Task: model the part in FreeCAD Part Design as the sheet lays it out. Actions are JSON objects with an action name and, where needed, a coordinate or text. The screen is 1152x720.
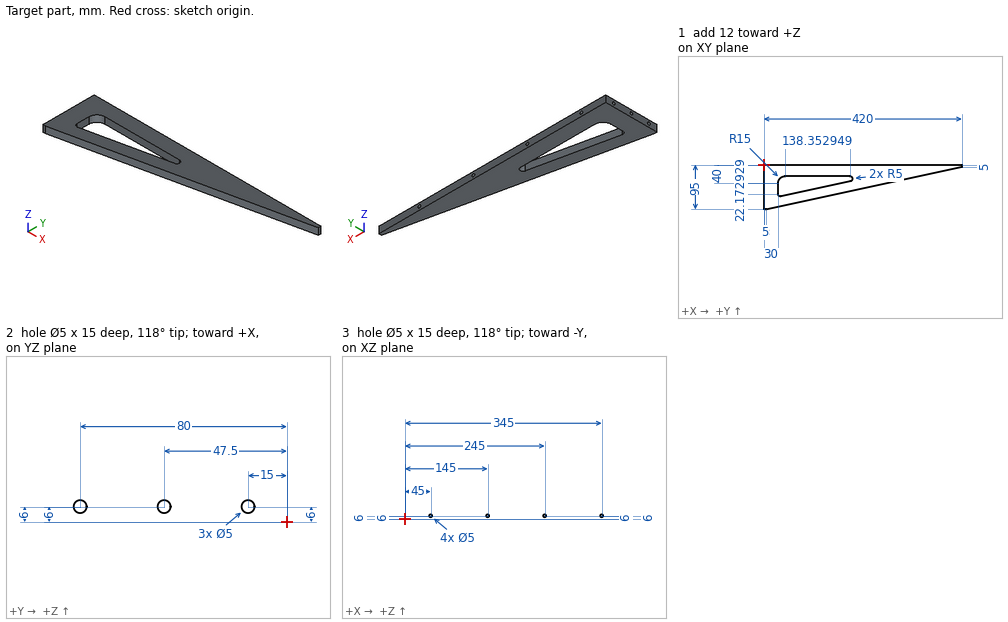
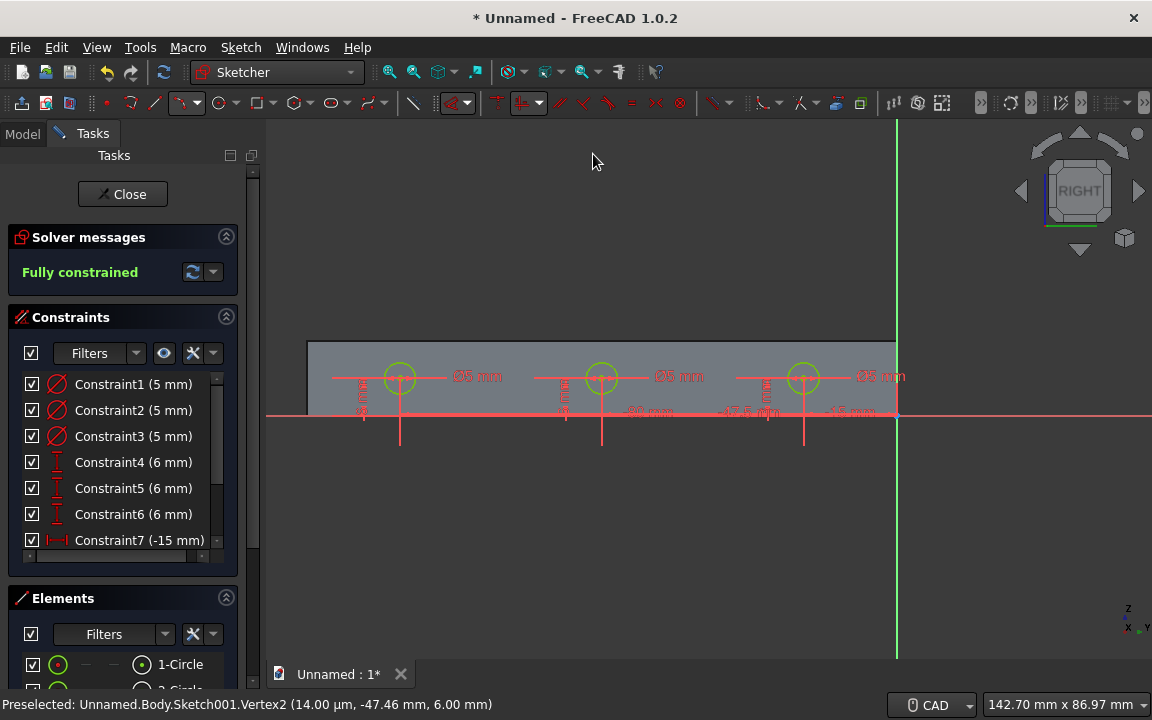
{"action": "left_click", "coordinate": [123, 194]}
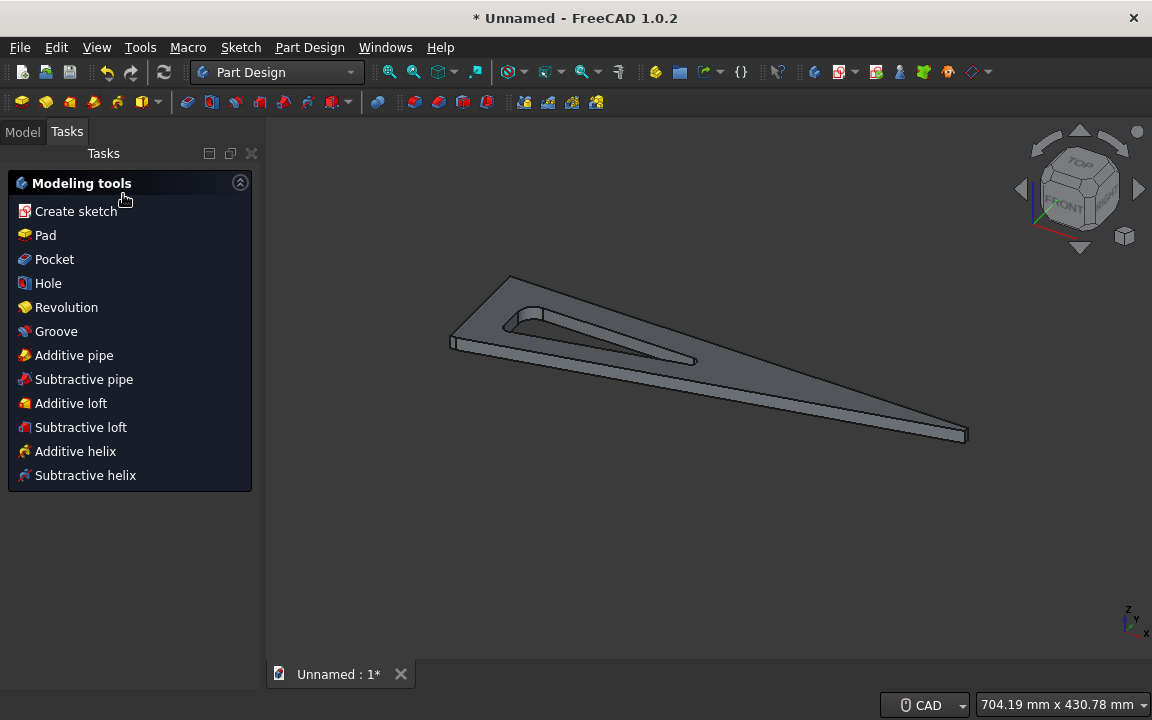
{"action": "left_click", "coordinate": [212, 102]}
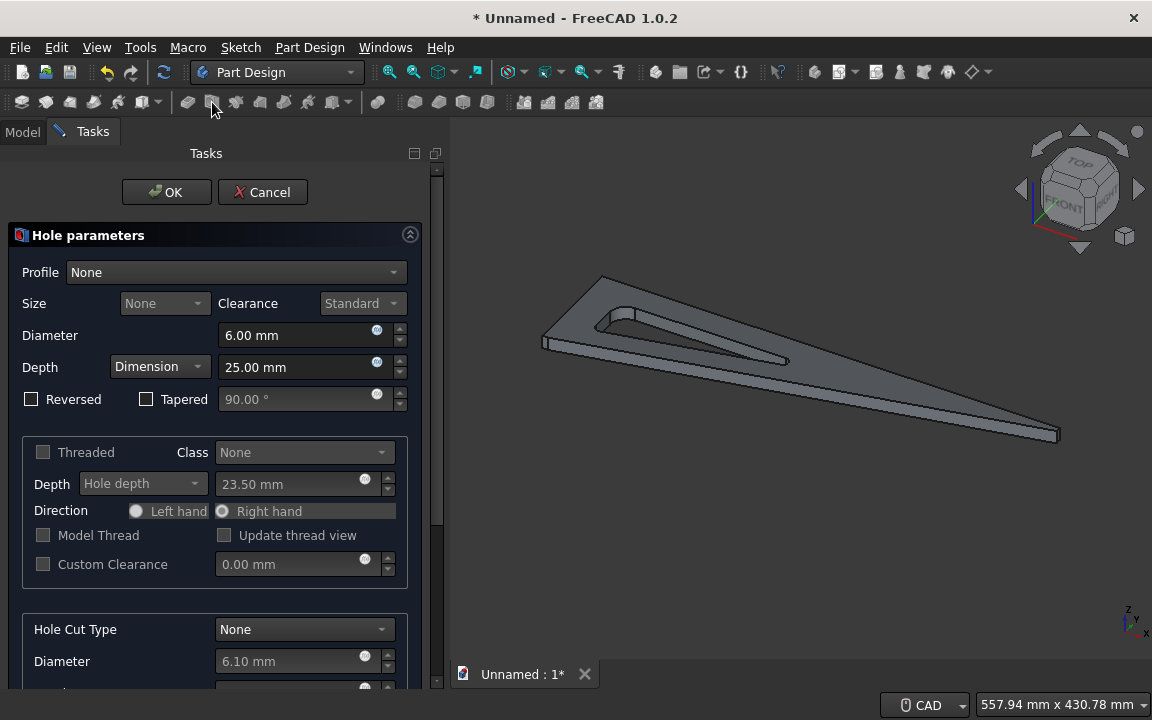
{"action": "triple_click", "coordinate": [305, 335]}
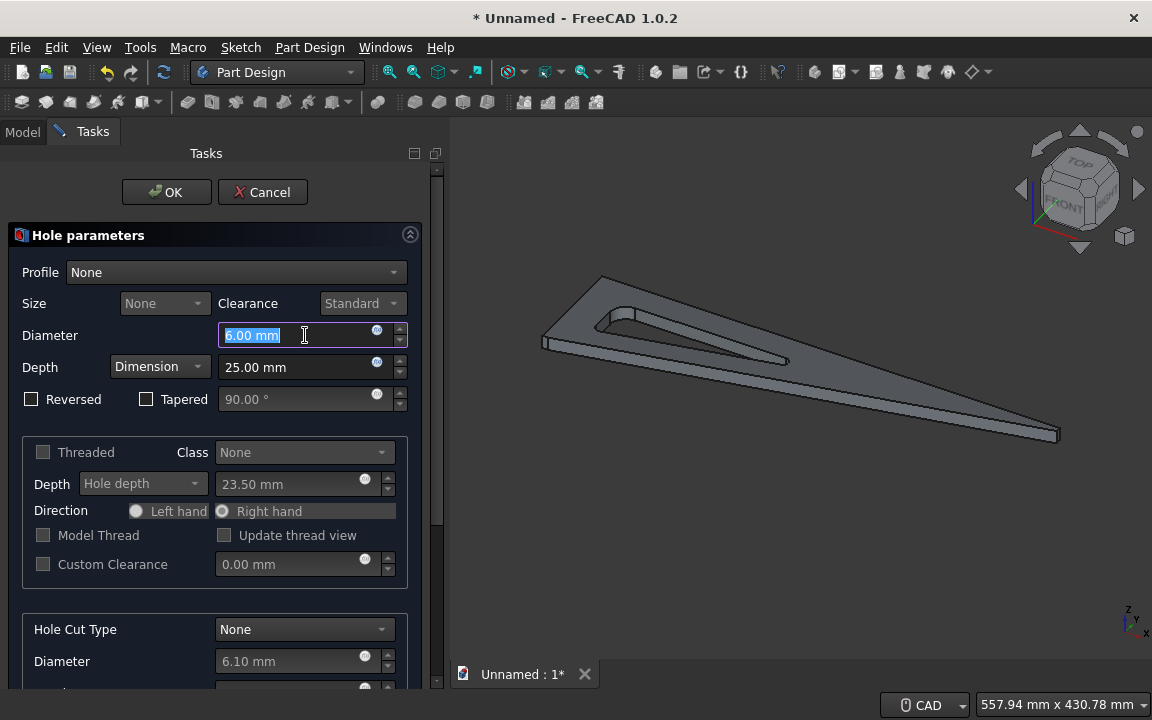
{"action": "type", "text": "5"}
{"action": "key", "text": "Tab"}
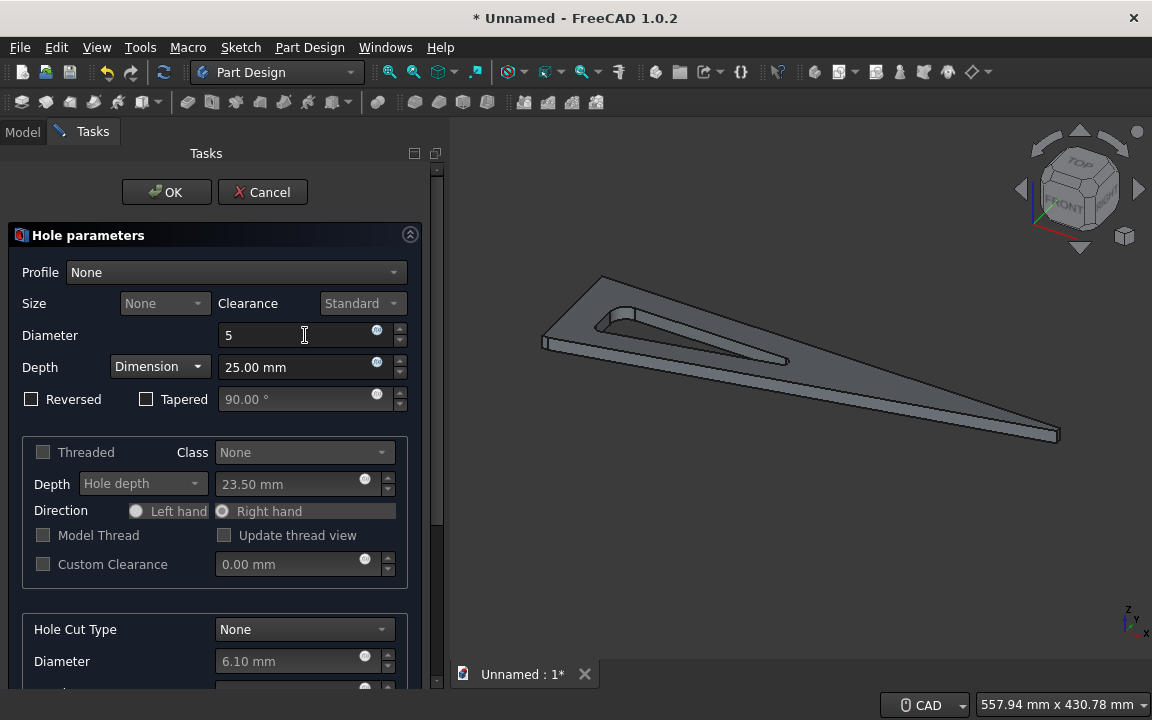
{"action": "triple_click", "coordinate": [305, 367]}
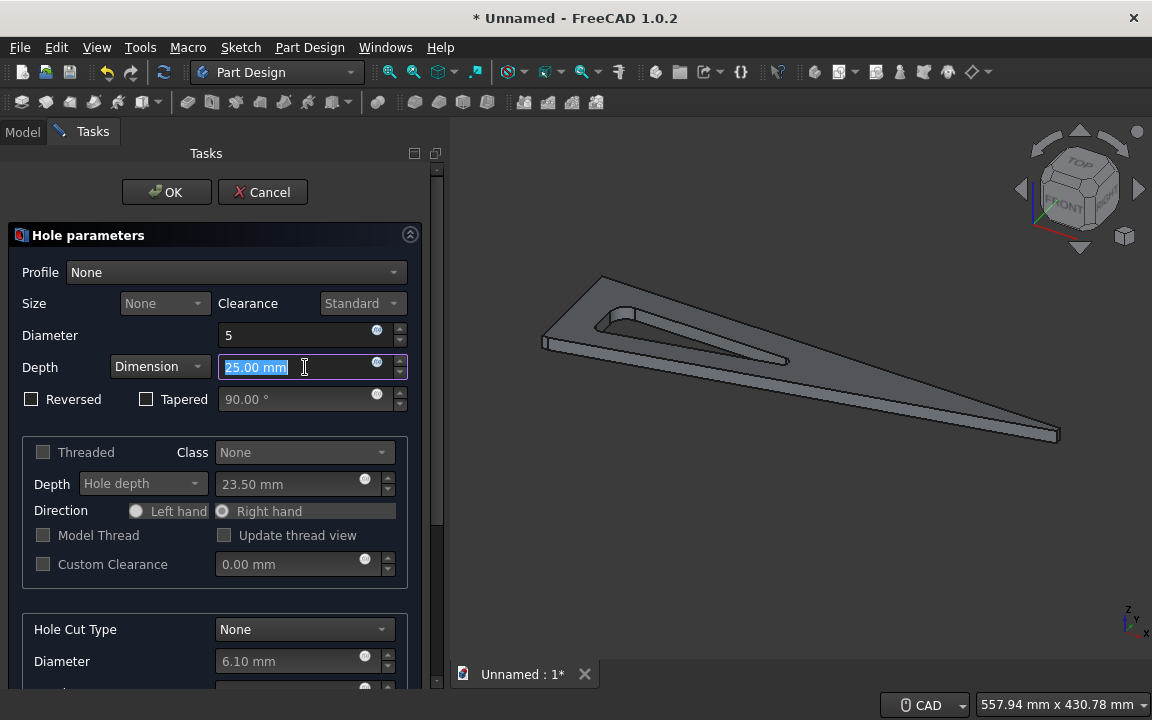
{"action": "type", "text": "15"}
{"action": "key", "text": "Tab"}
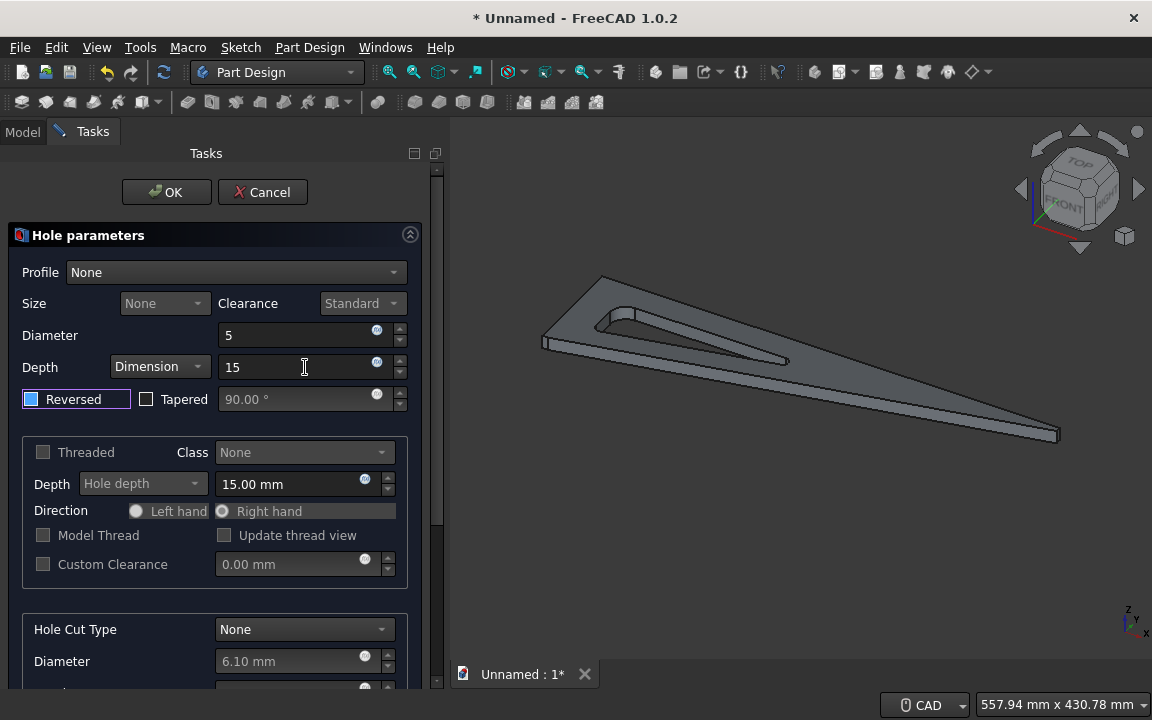
{"action": "left_click", "coordinate": [30, 399]}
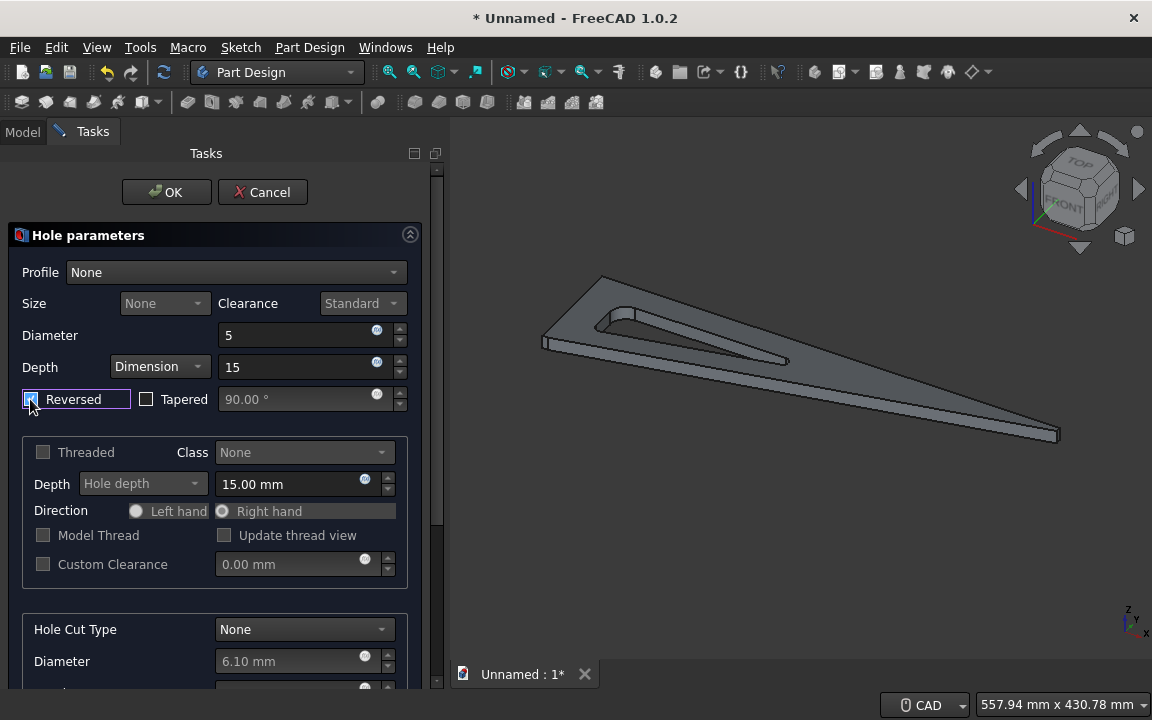
{"action": "left_click", "coordinate": [167, 192]}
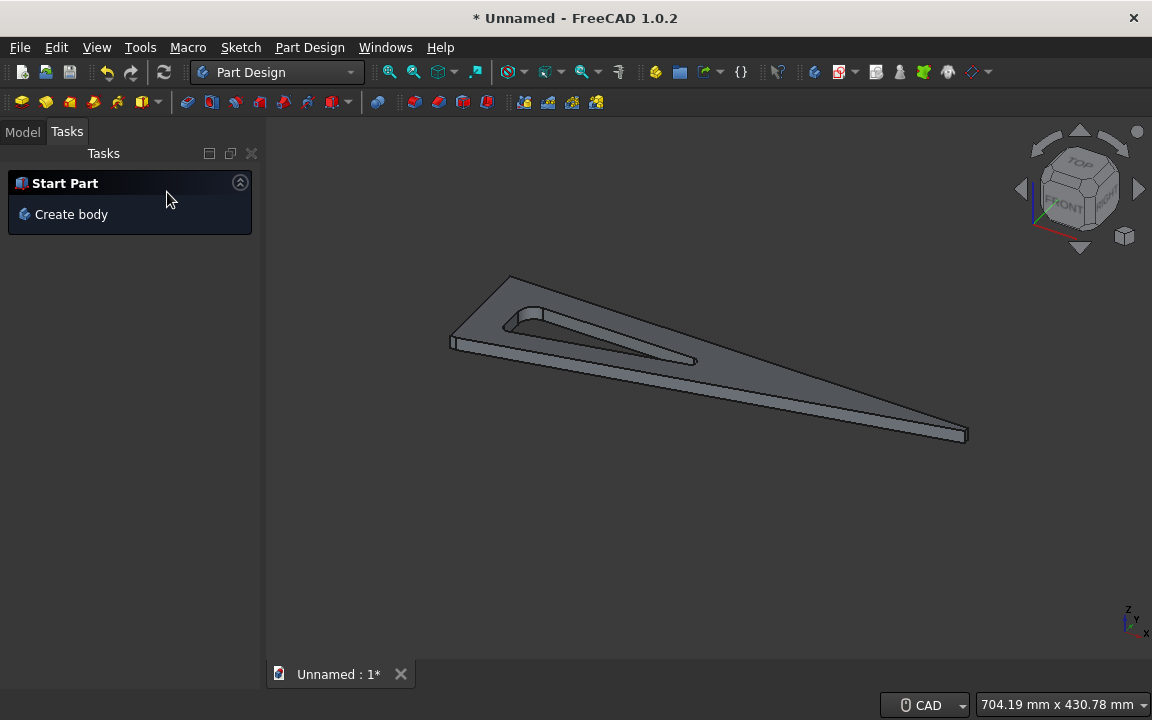
{"action": "left_click", "coordinate": [840, 72]}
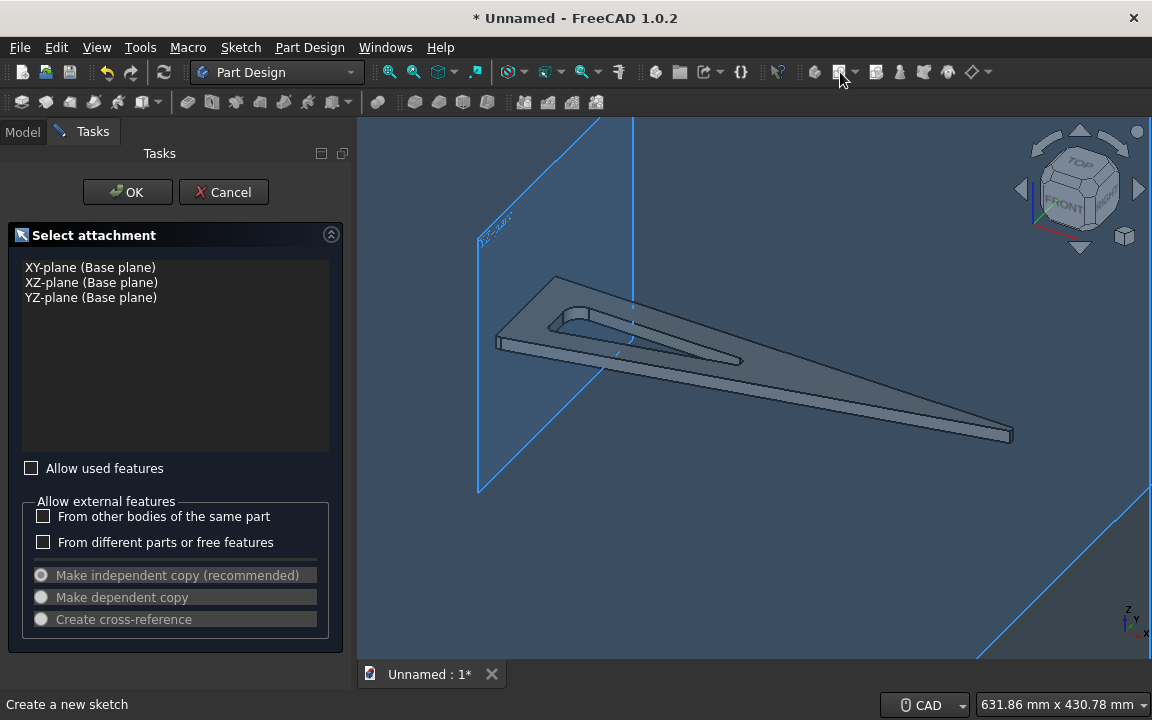
{"action": "left_click", "coordinate": [82, 282]}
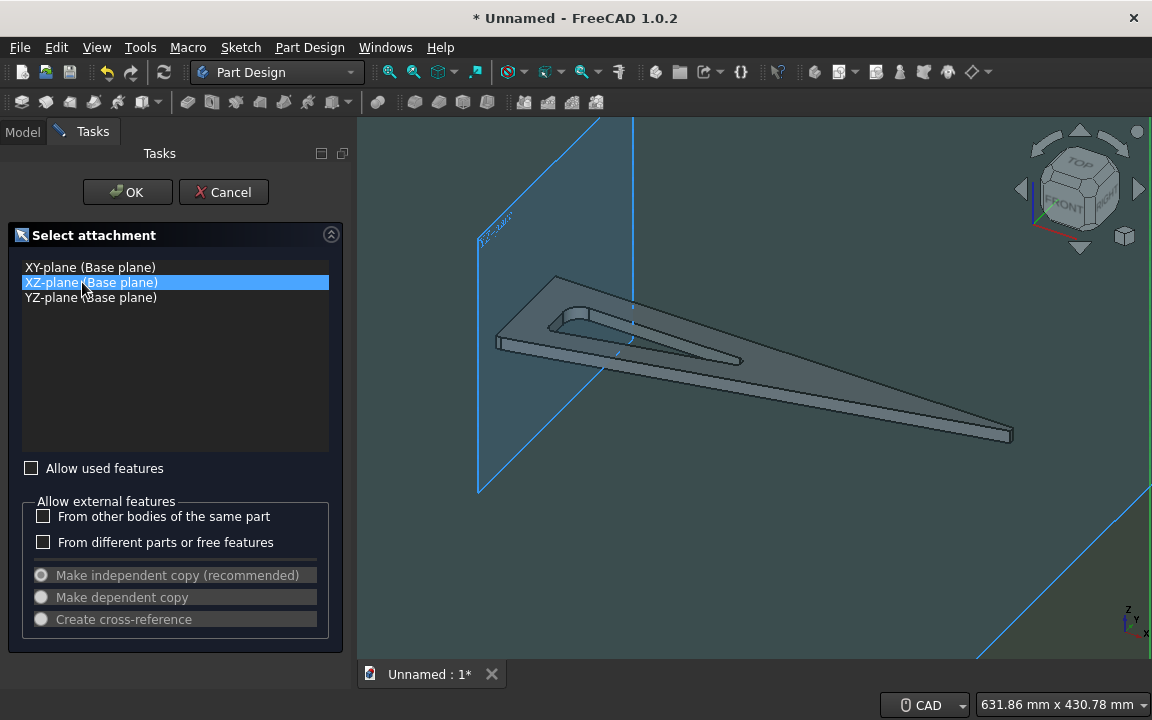
{"action": "left_click", "coordinate": [128, 192]}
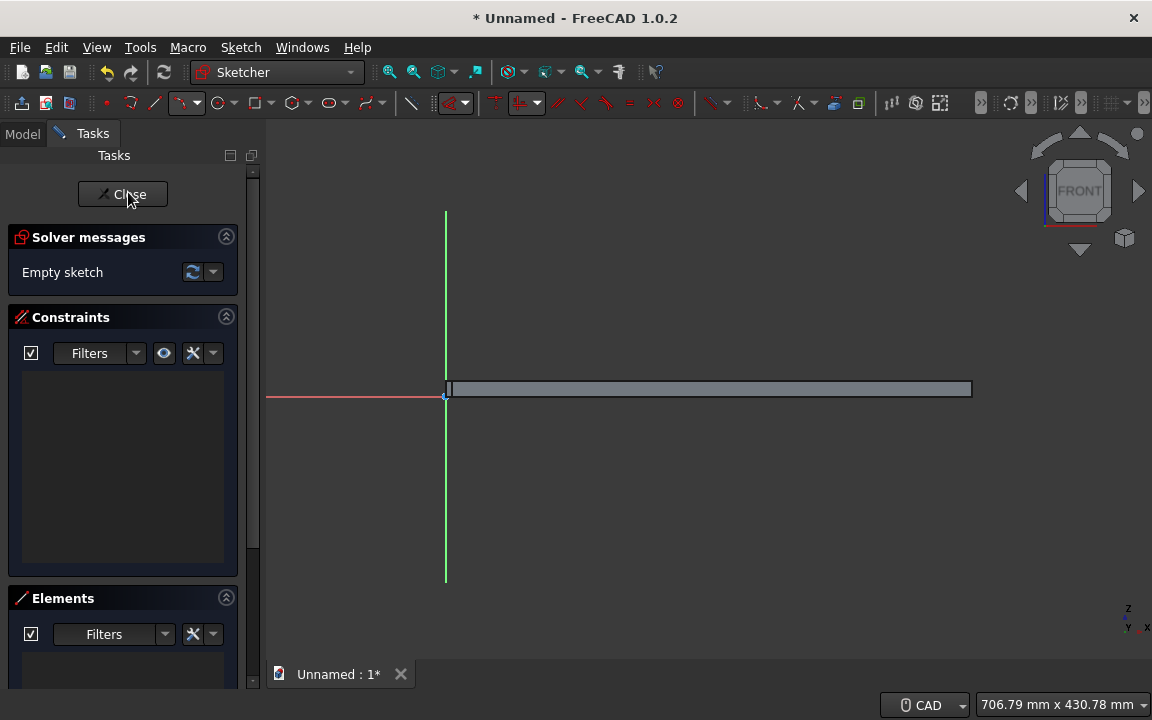
{"action": "left_click", "coordinate": [70, 104]}